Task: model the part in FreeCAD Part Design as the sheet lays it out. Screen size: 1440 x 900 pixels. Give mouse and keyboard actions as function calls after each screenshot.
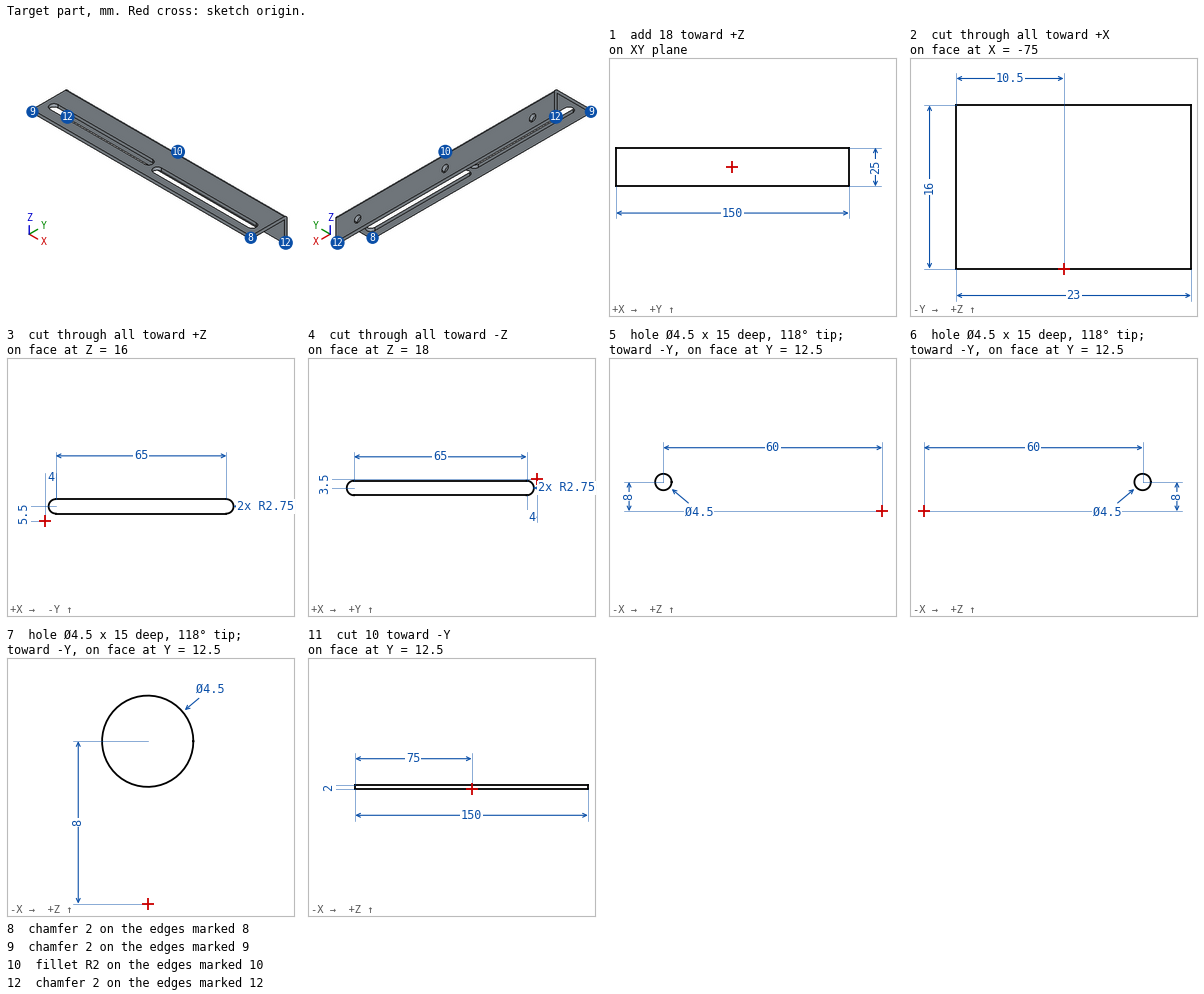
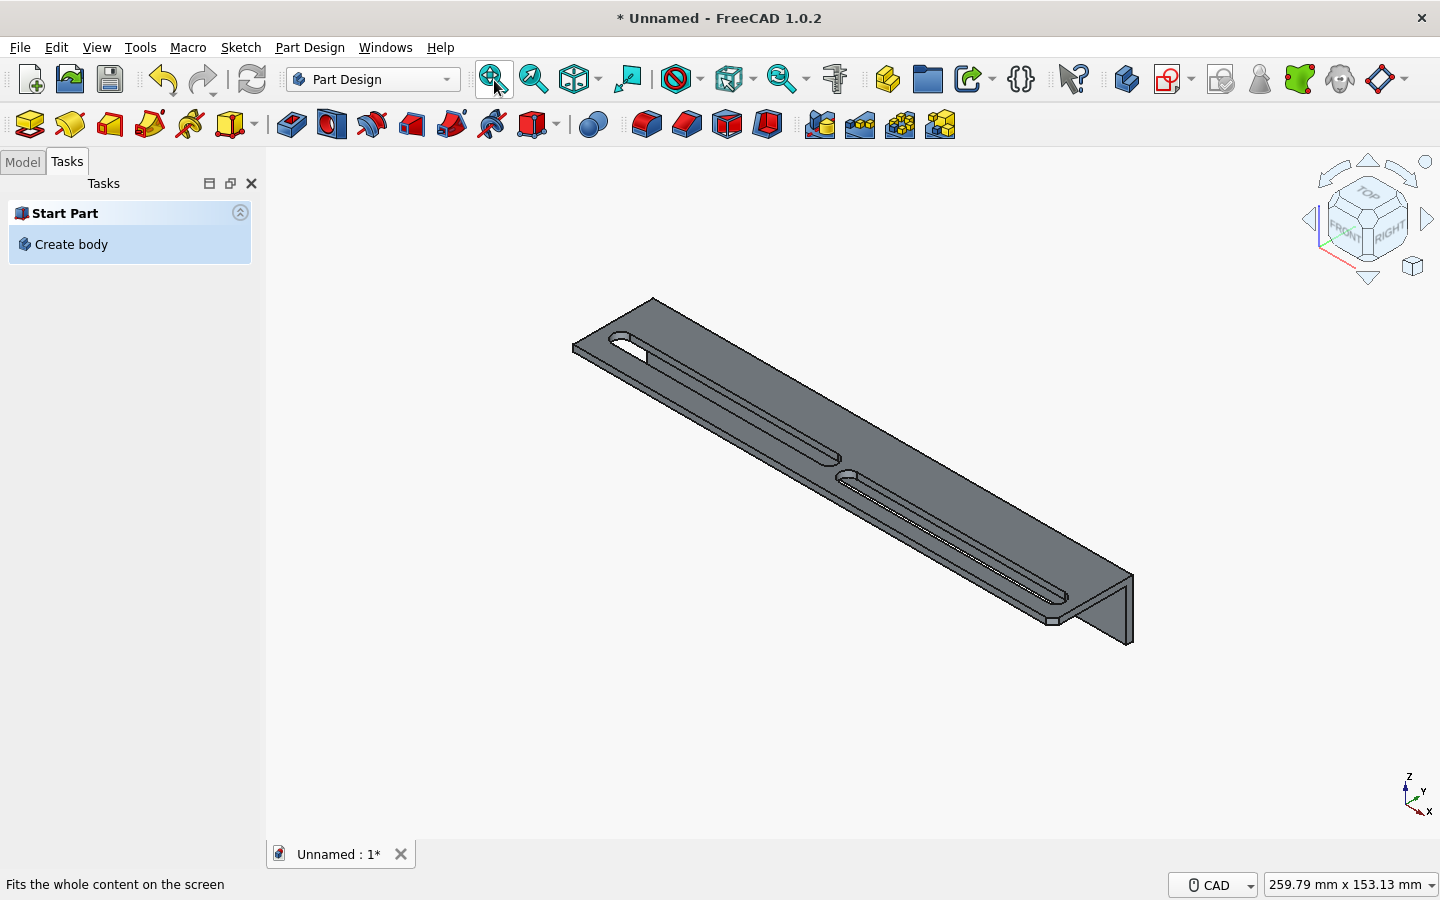
key(2)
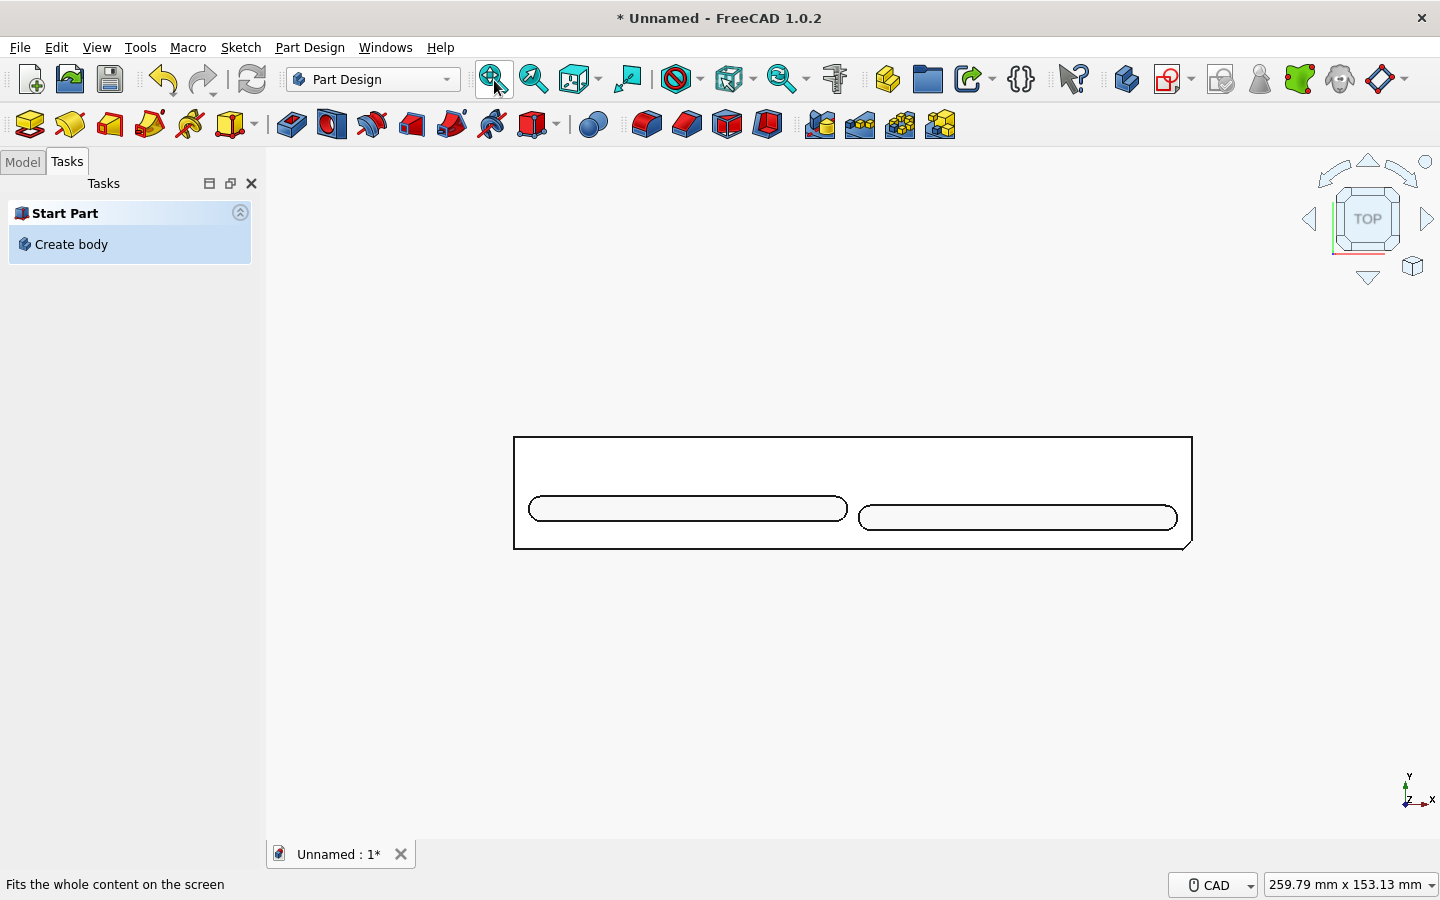
scroll(514, 548, up, 8)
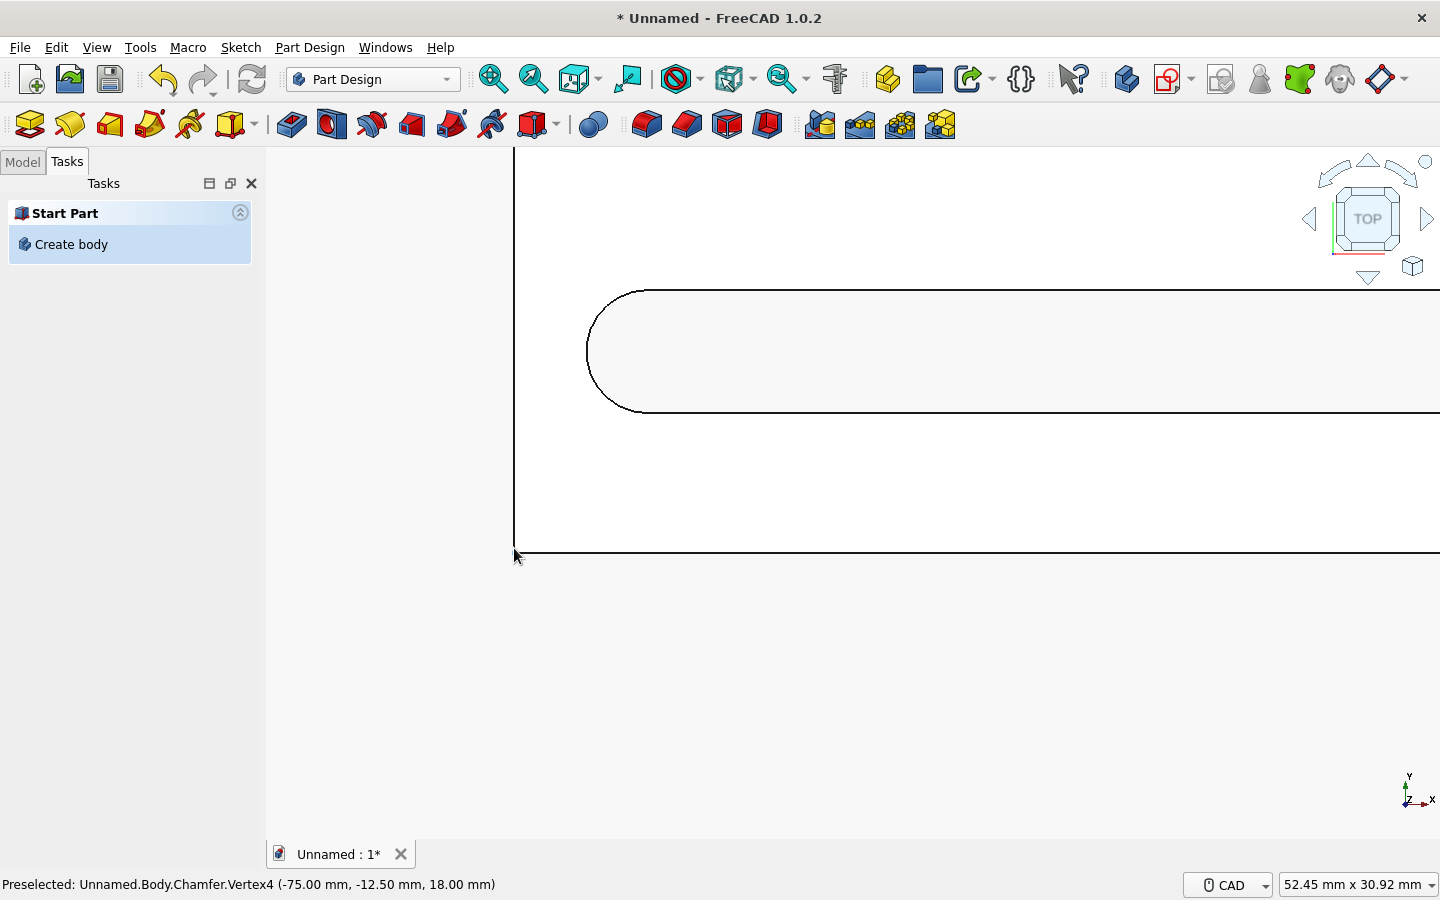
click(494, 80)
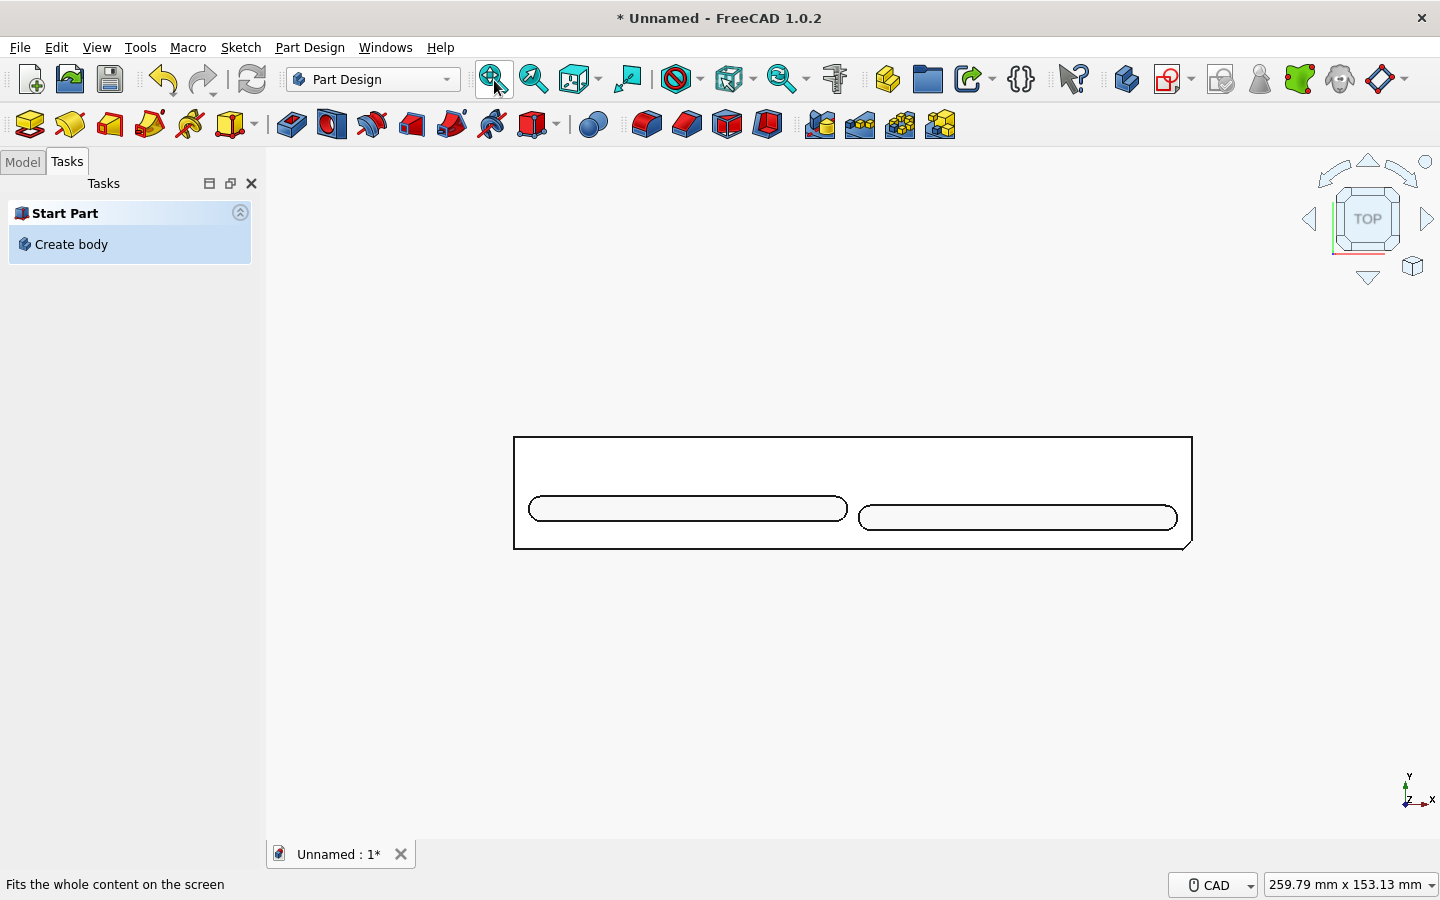
key(0)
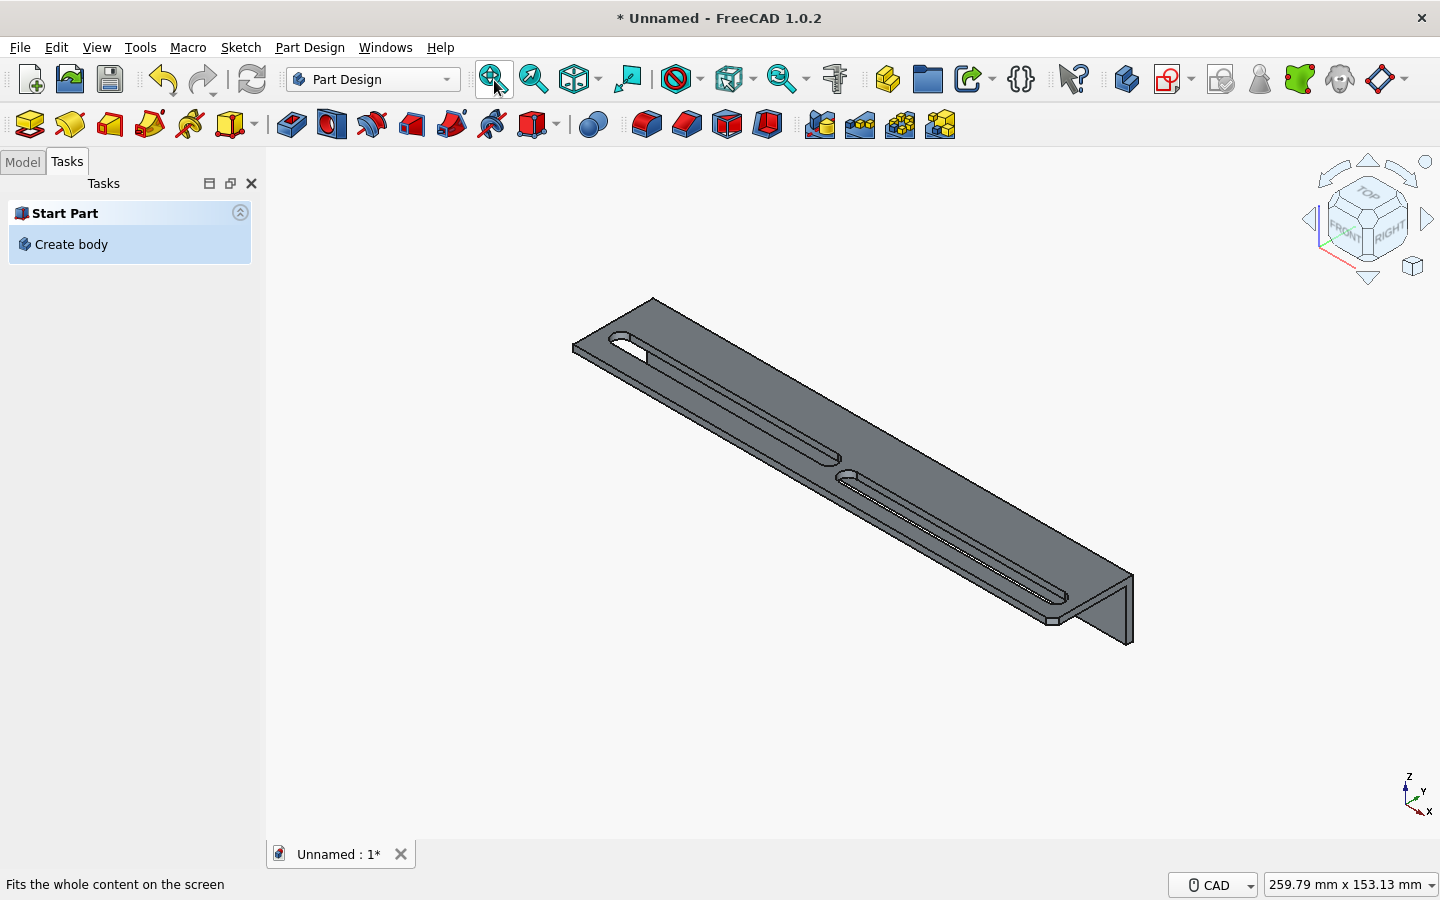
scroll(573, 347, up, 8)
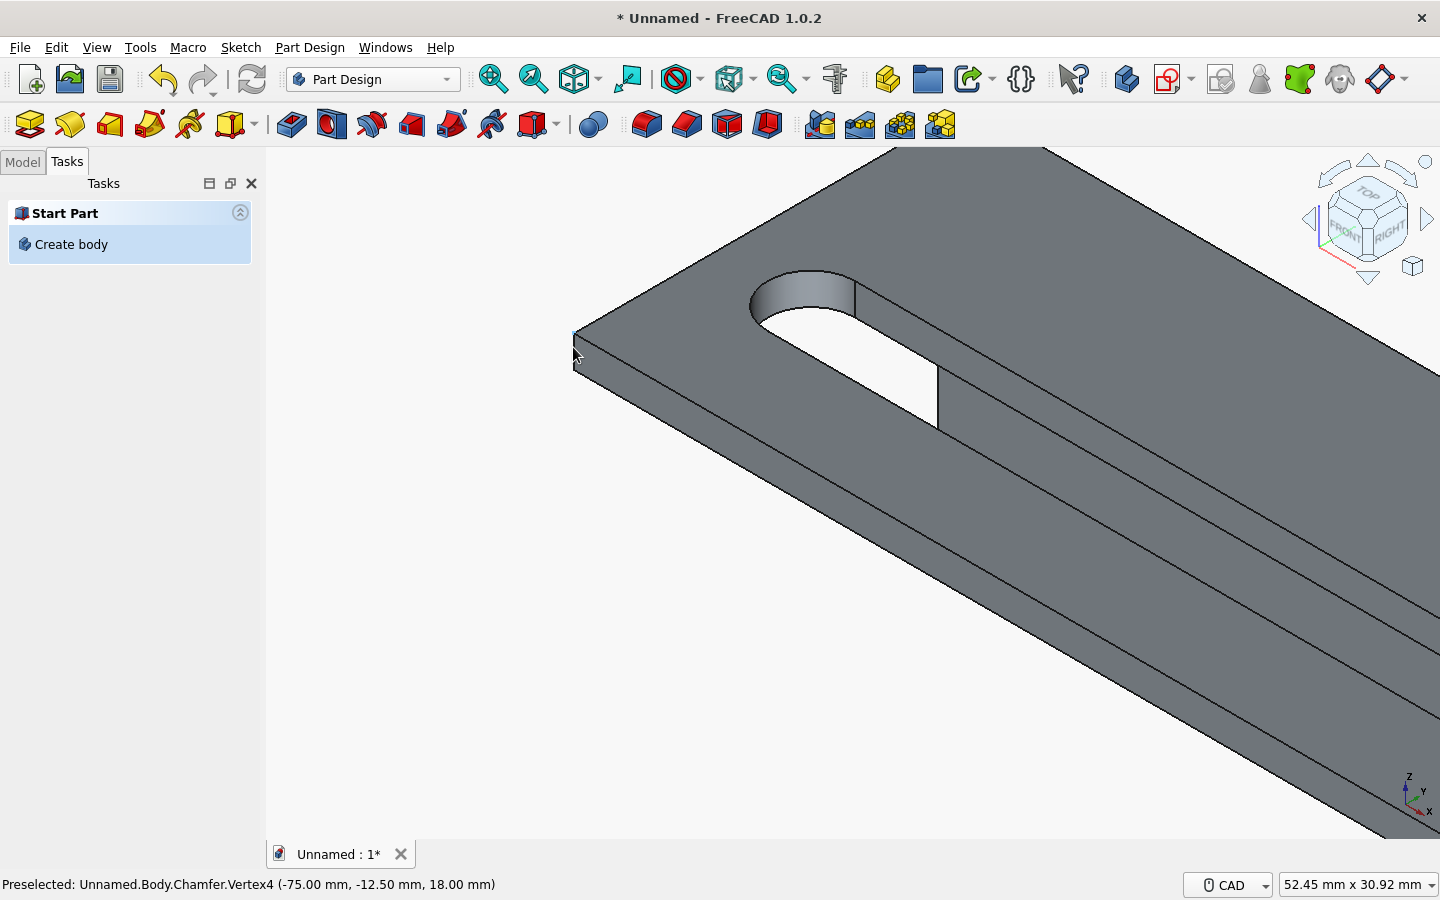
click(494, 80)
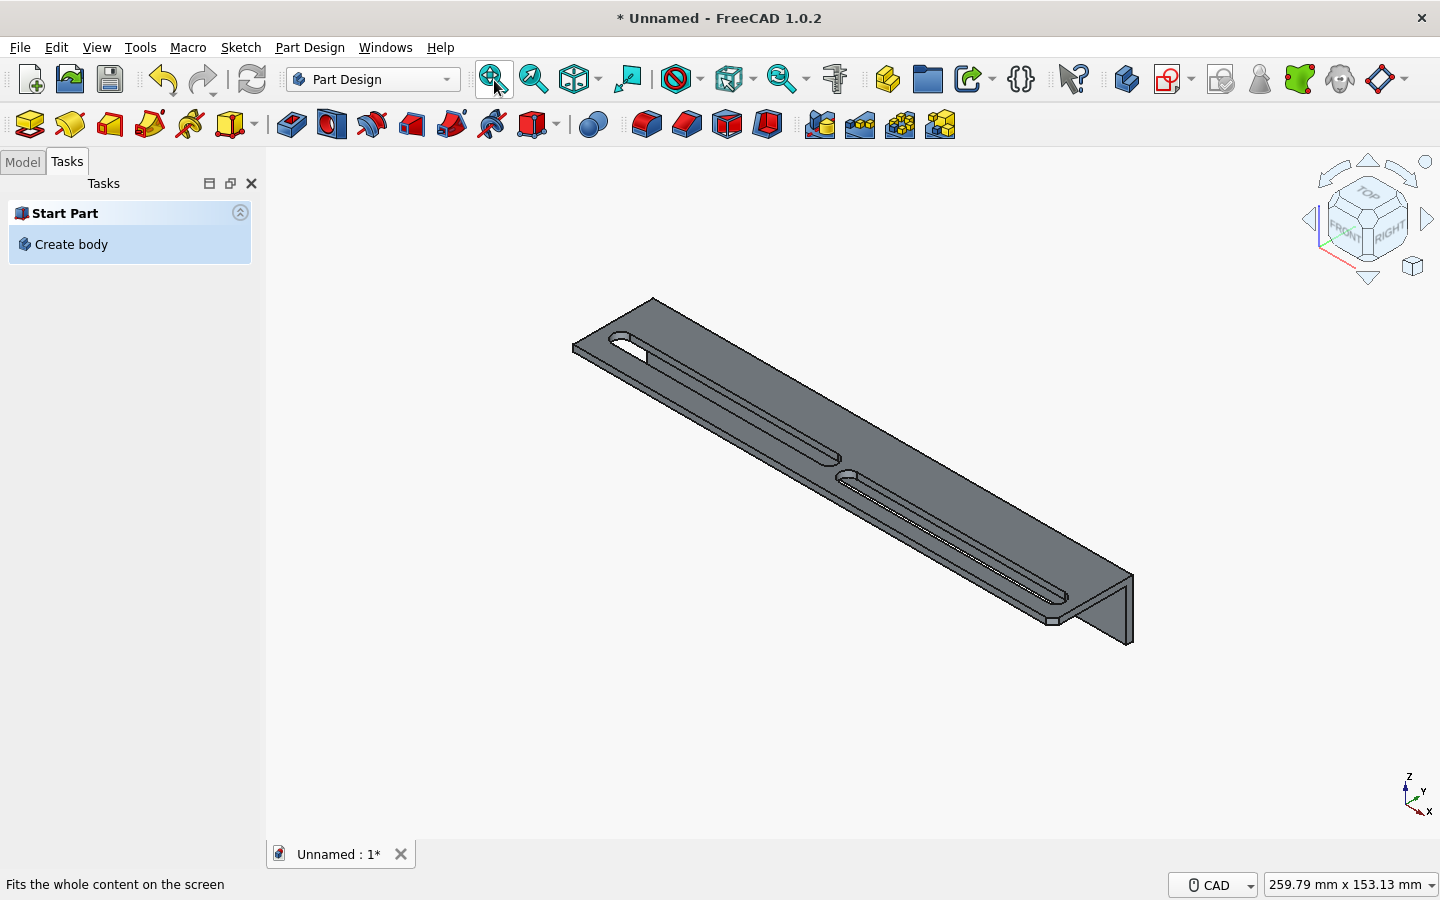
key(1)